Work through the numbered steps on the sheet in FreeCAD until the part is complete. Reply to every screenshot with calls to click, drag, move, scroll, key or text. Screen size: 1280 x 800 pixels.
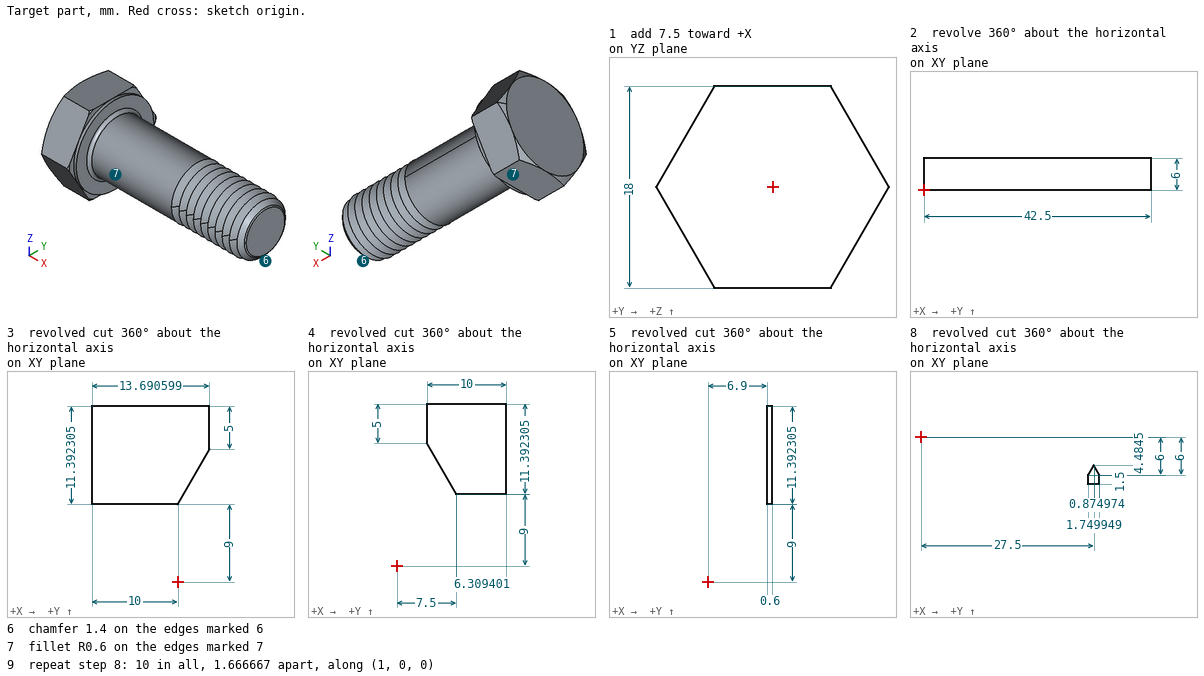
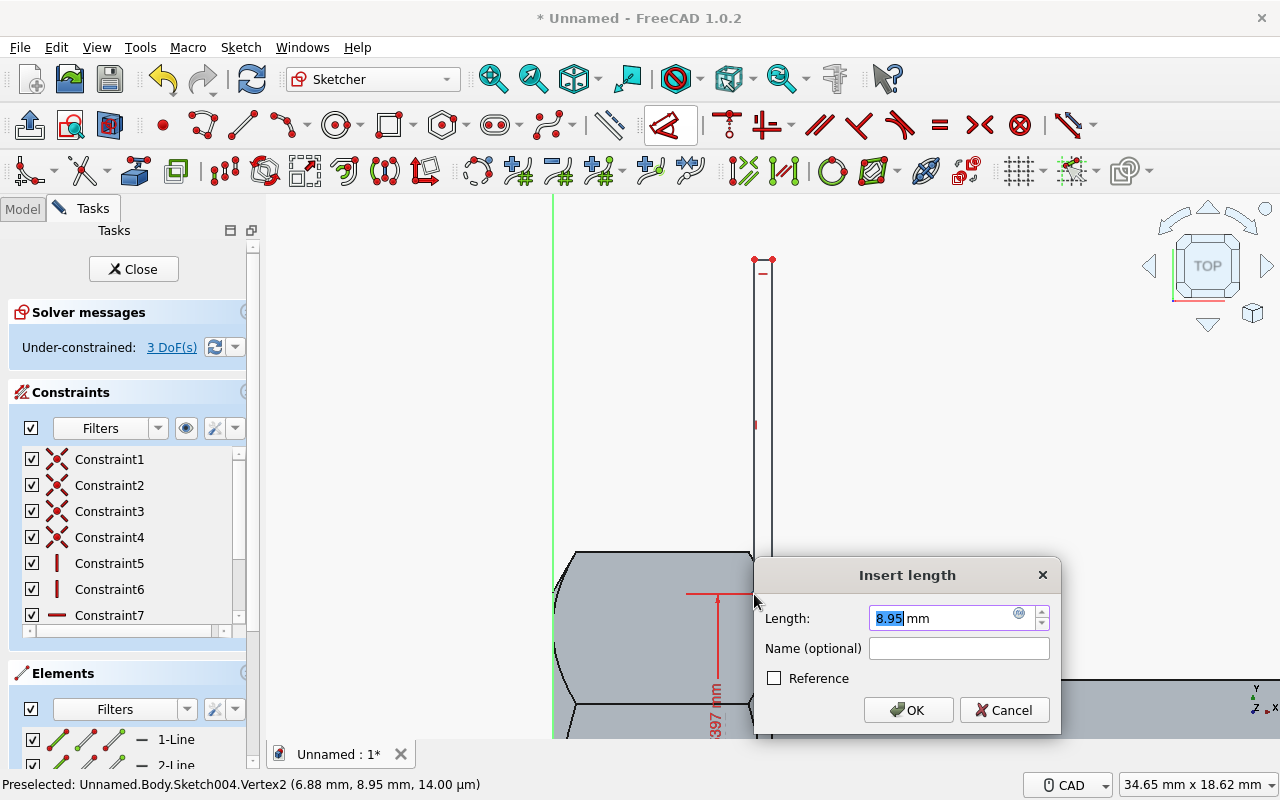
text(9)
key(Return)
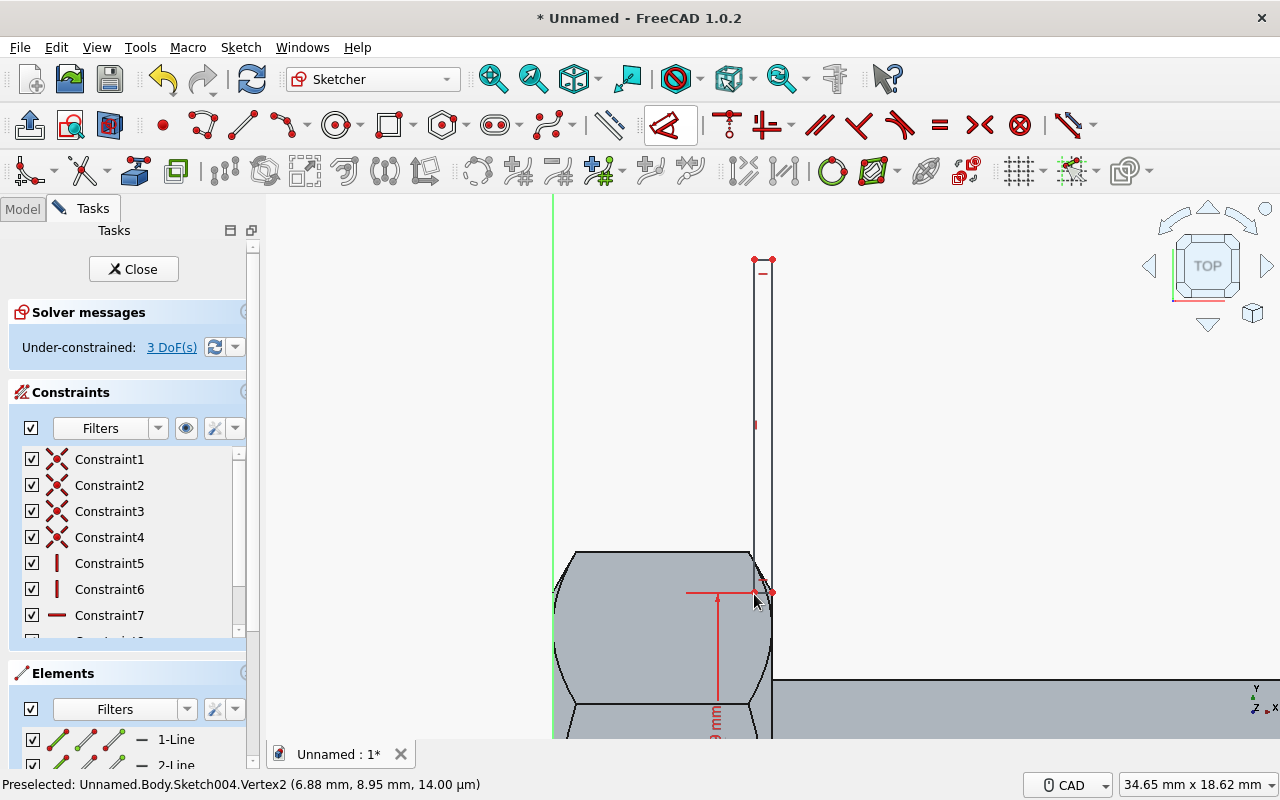
scroll(763, 593, up, 5)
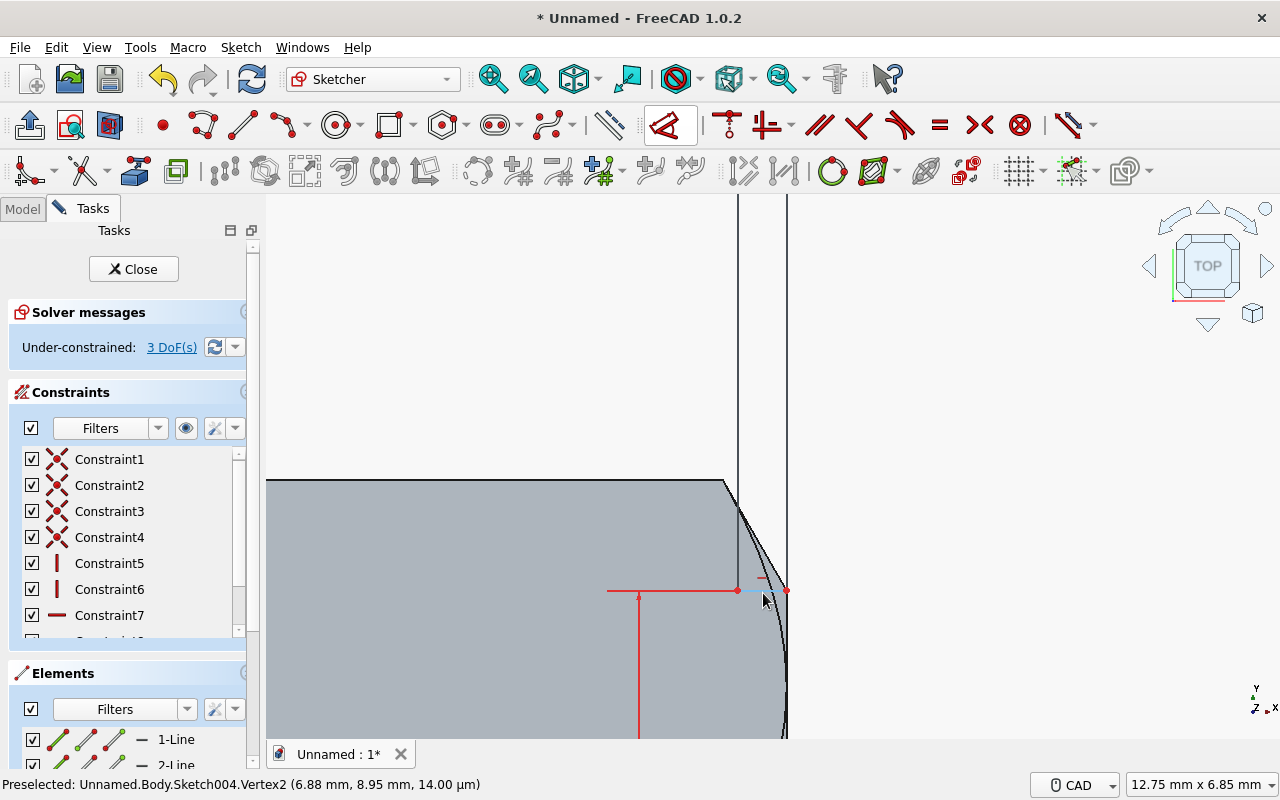
click(762, 591)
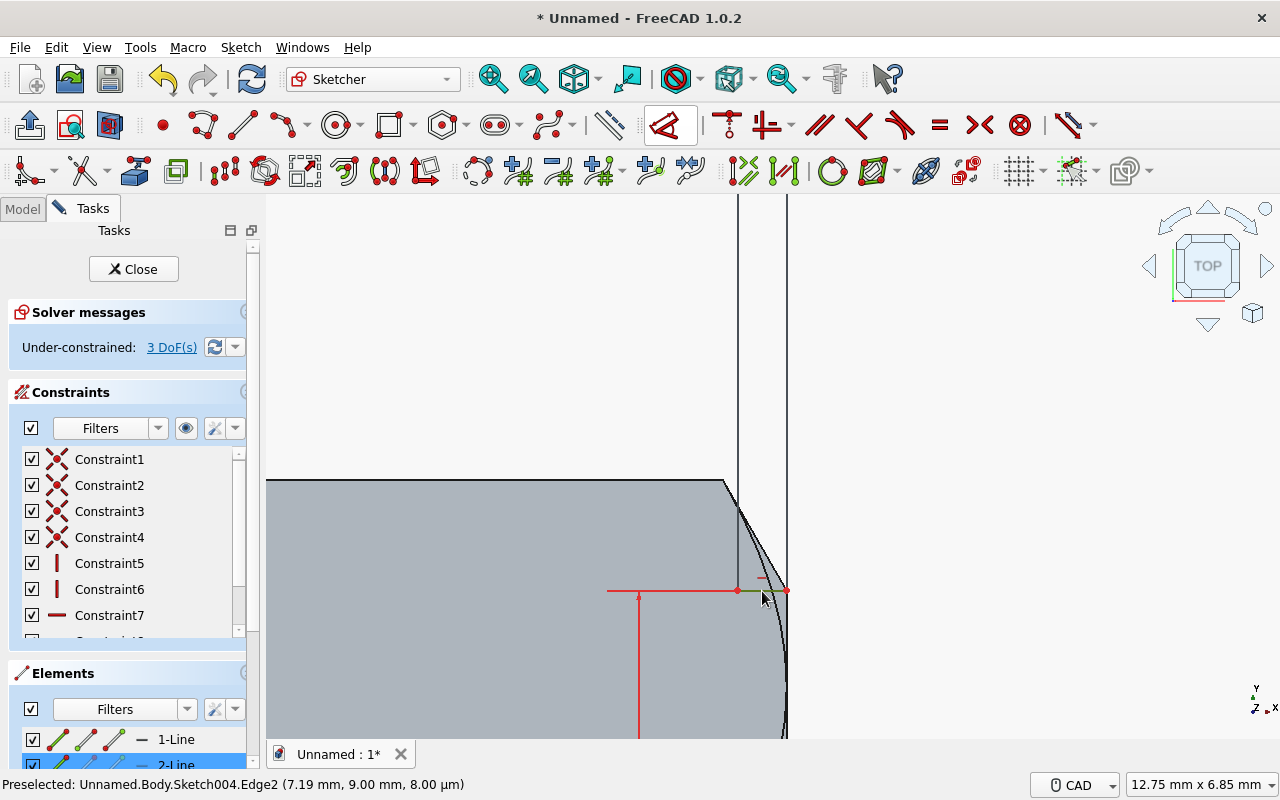
key(l)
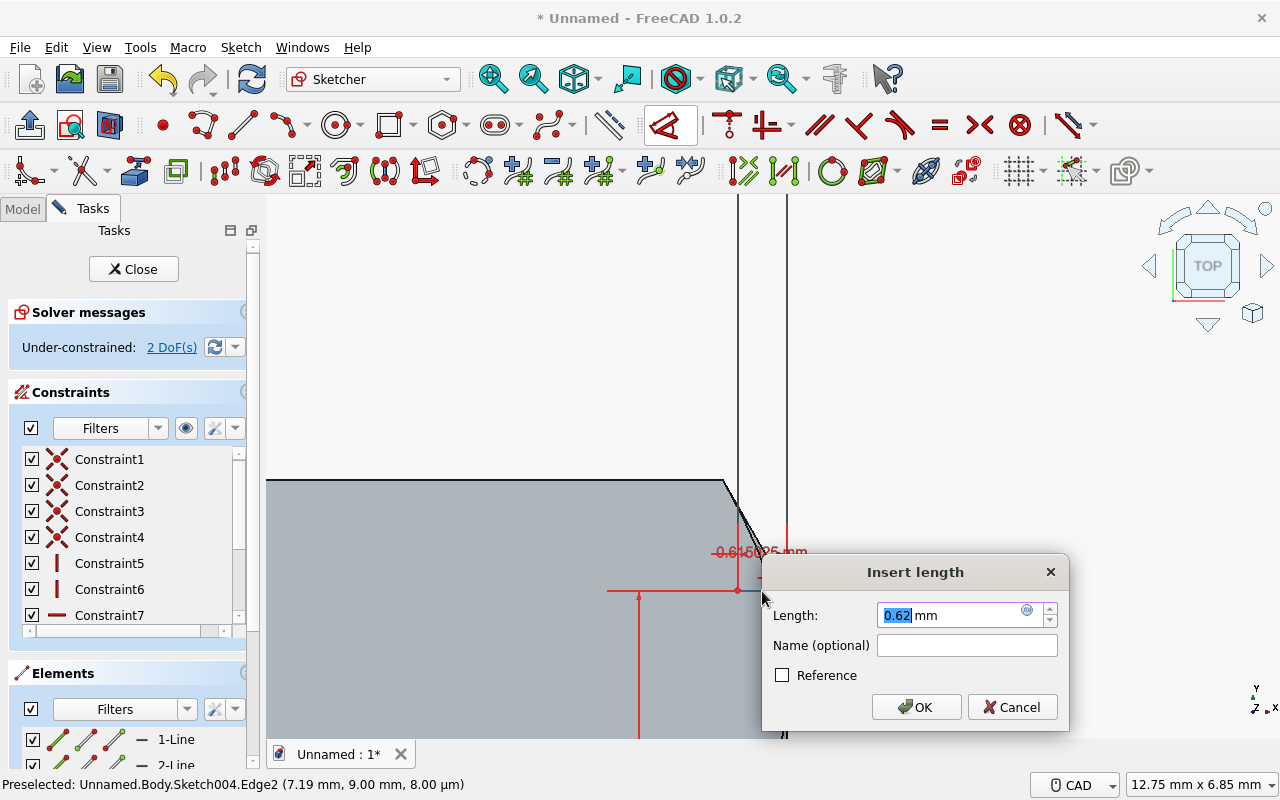
text(0.6)
key(Return)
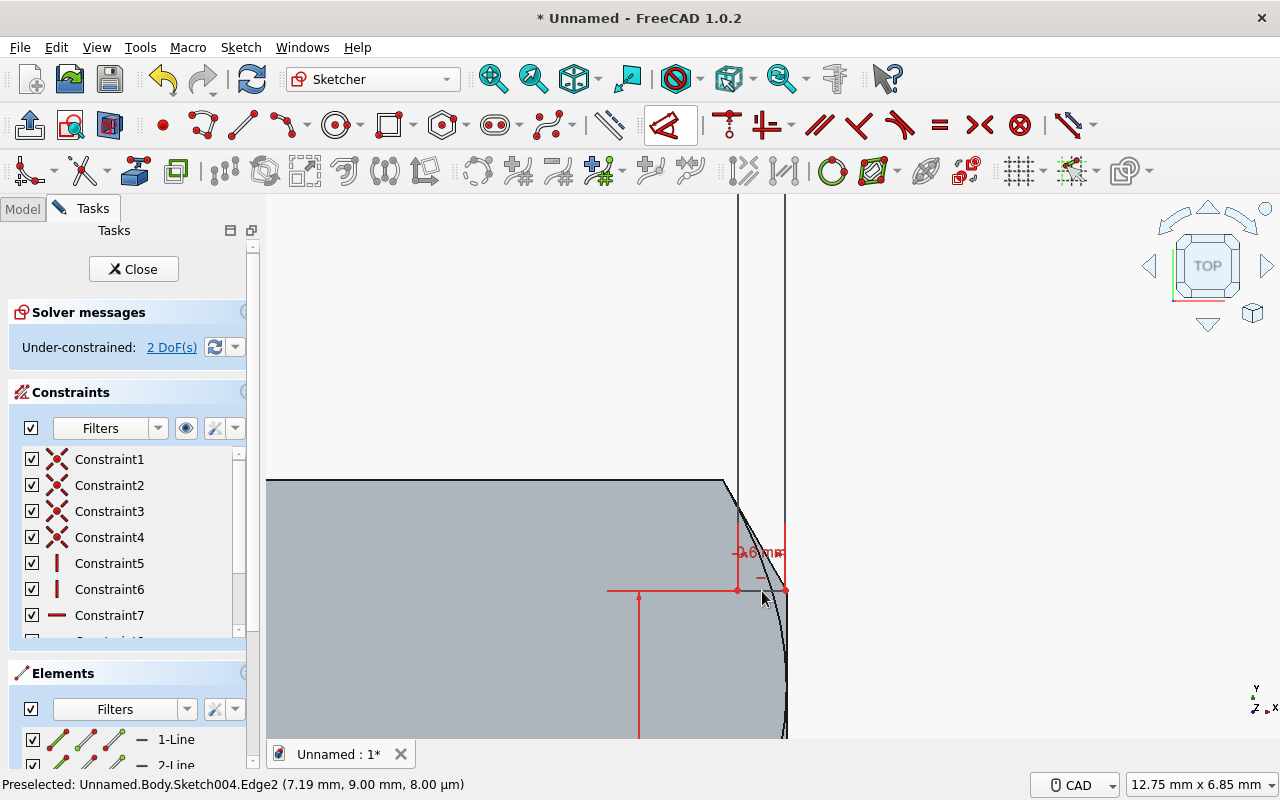
scroll(759, 459, down, 8)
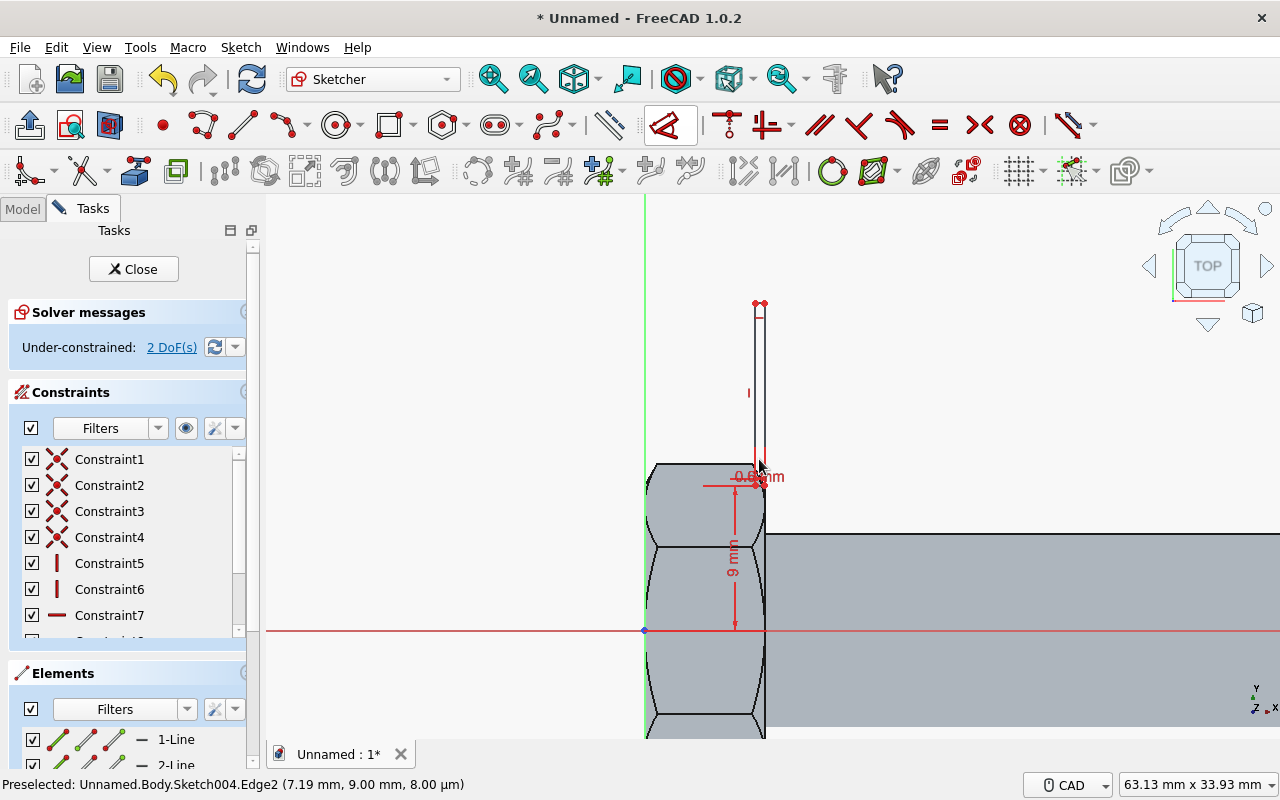
scroll(755, 303, up, 2)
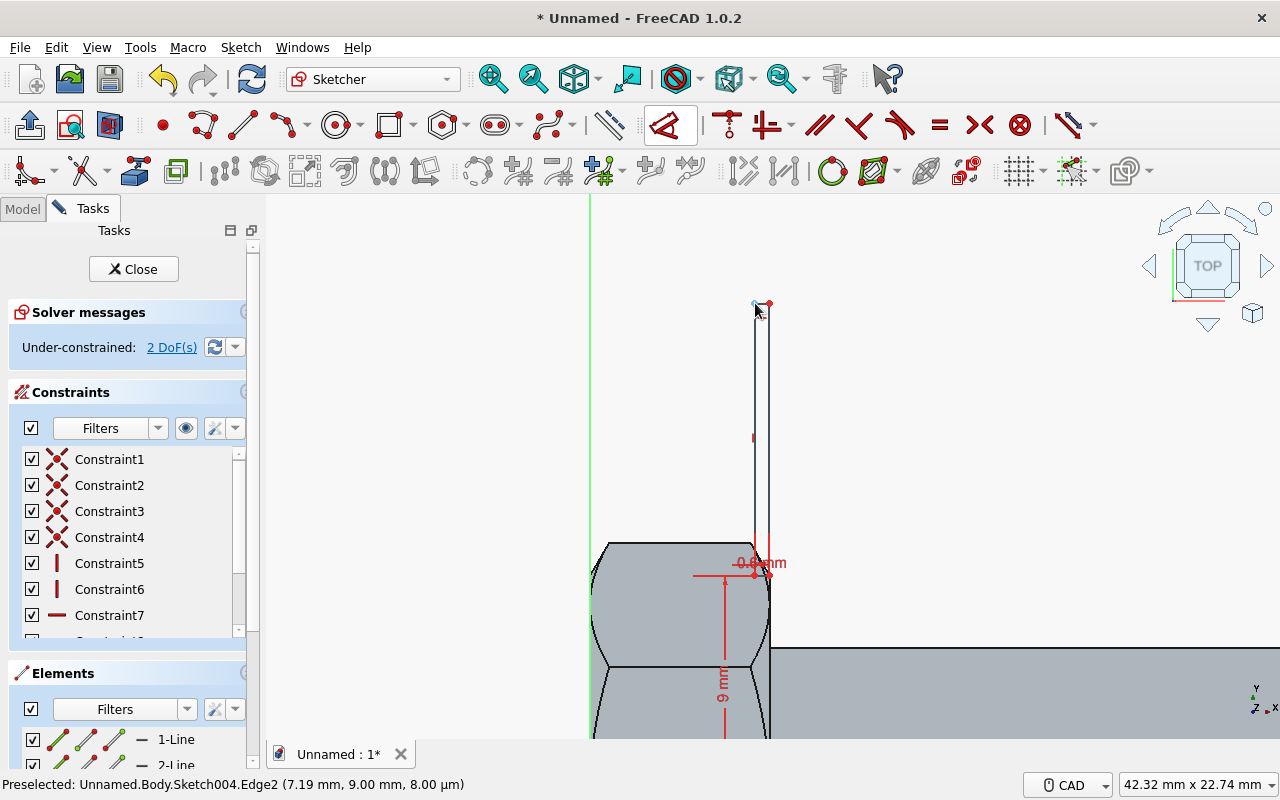
click(755, 304)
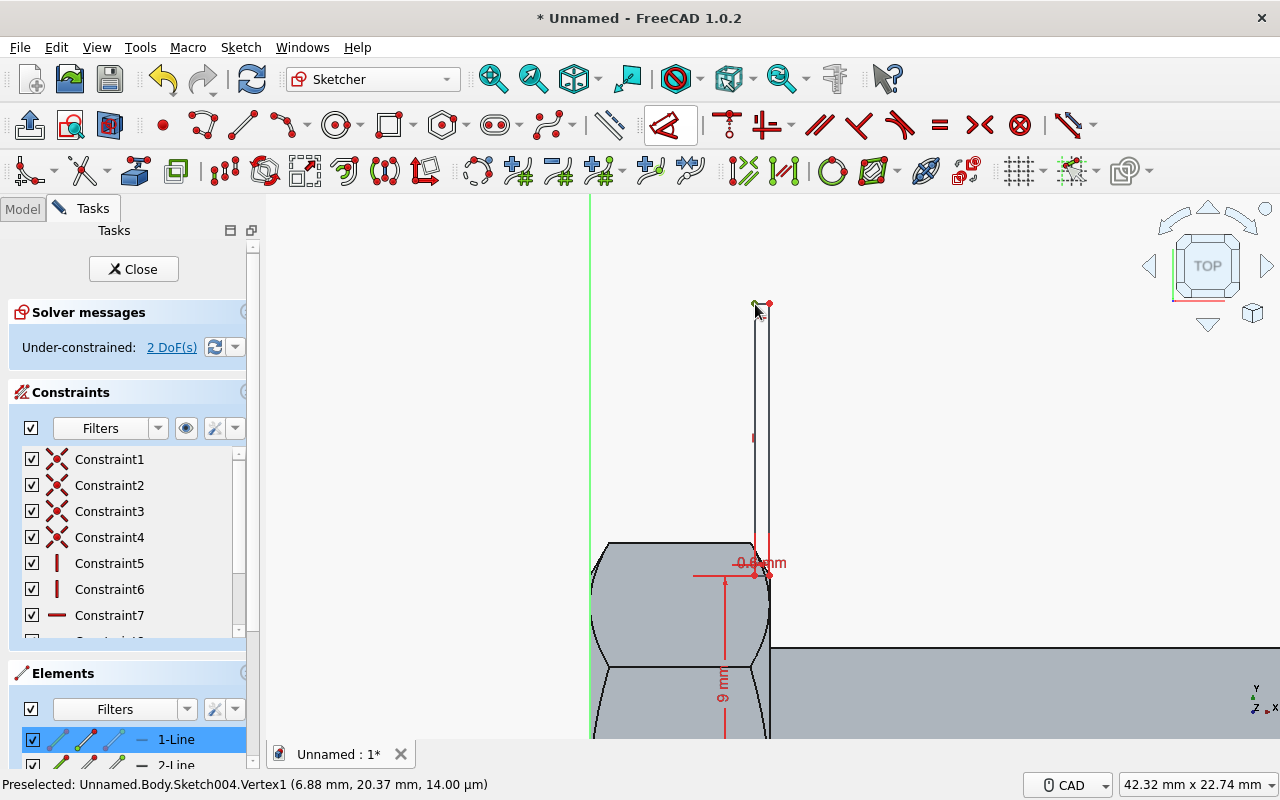
key(l)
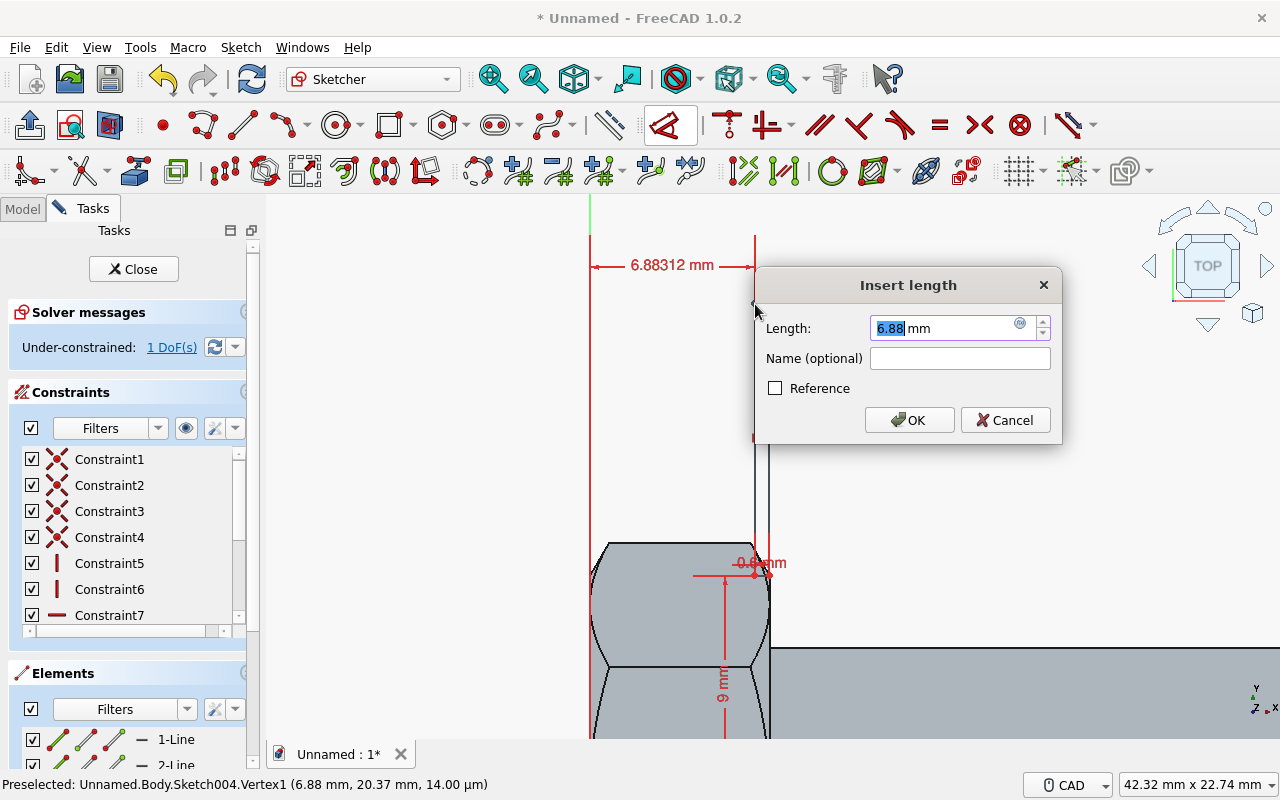
text(6.9)
key(Return)